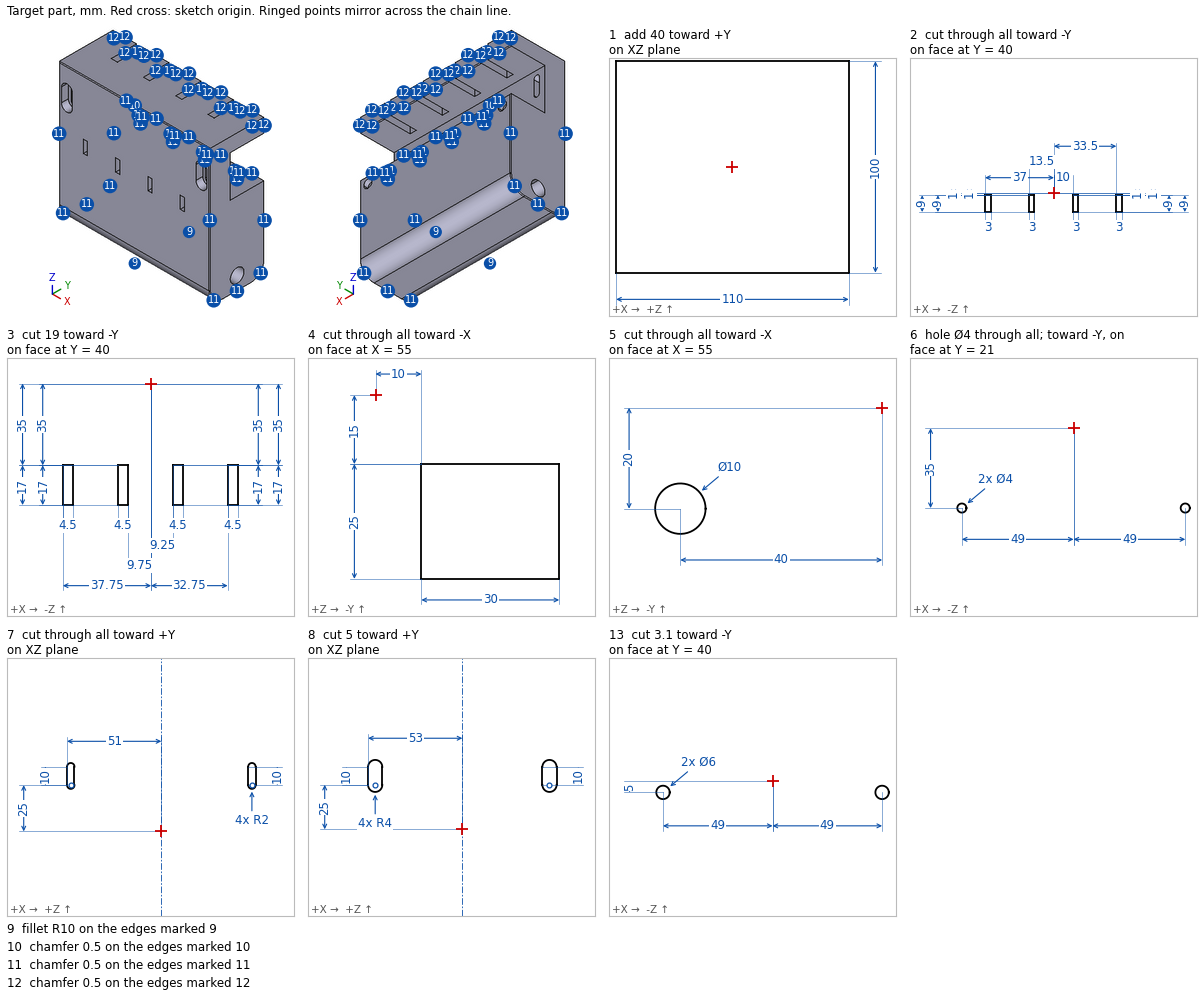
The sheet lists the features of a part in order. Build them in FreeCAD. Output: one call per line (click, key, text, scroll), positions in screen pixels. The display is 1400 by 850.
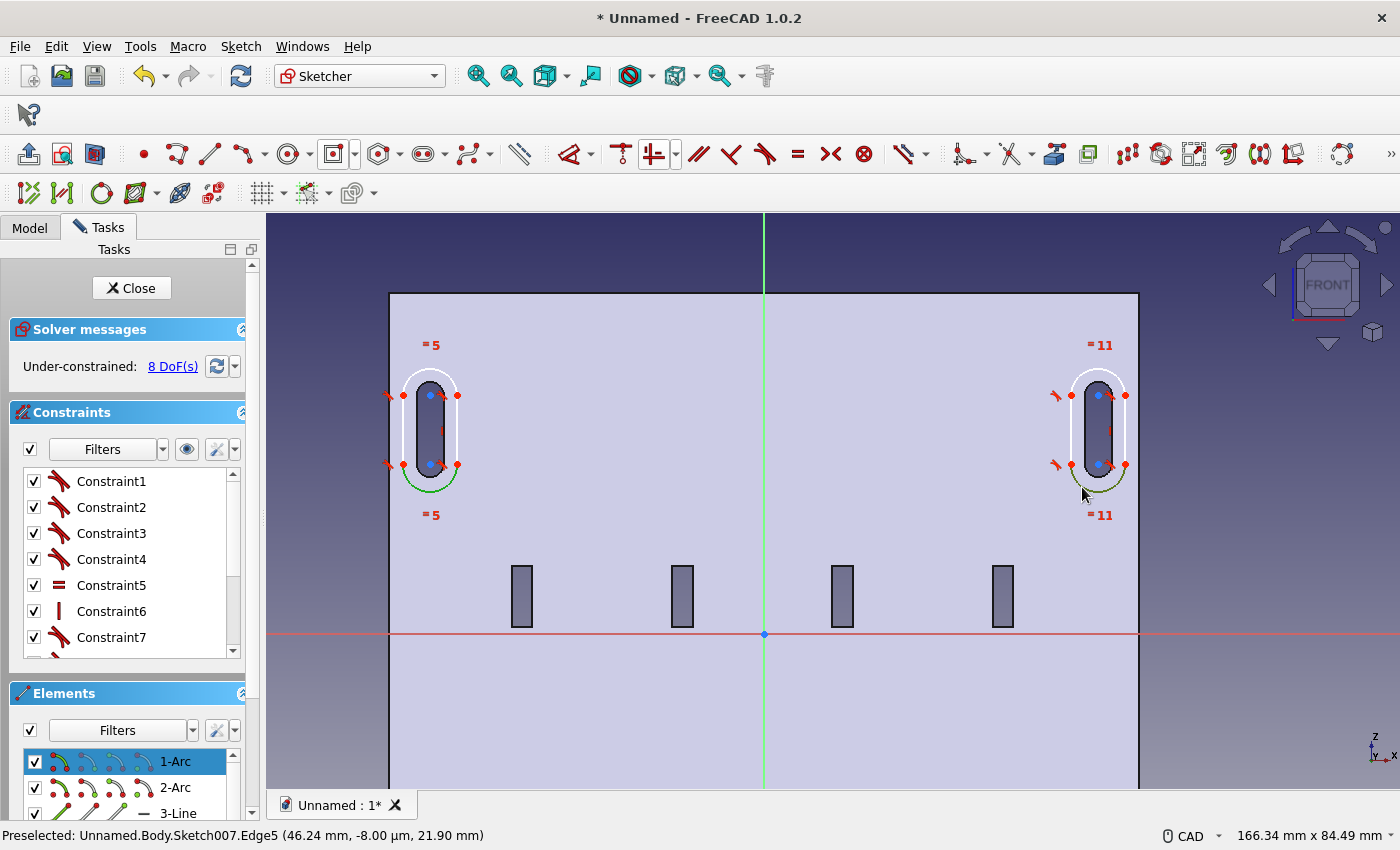
click(798, 154)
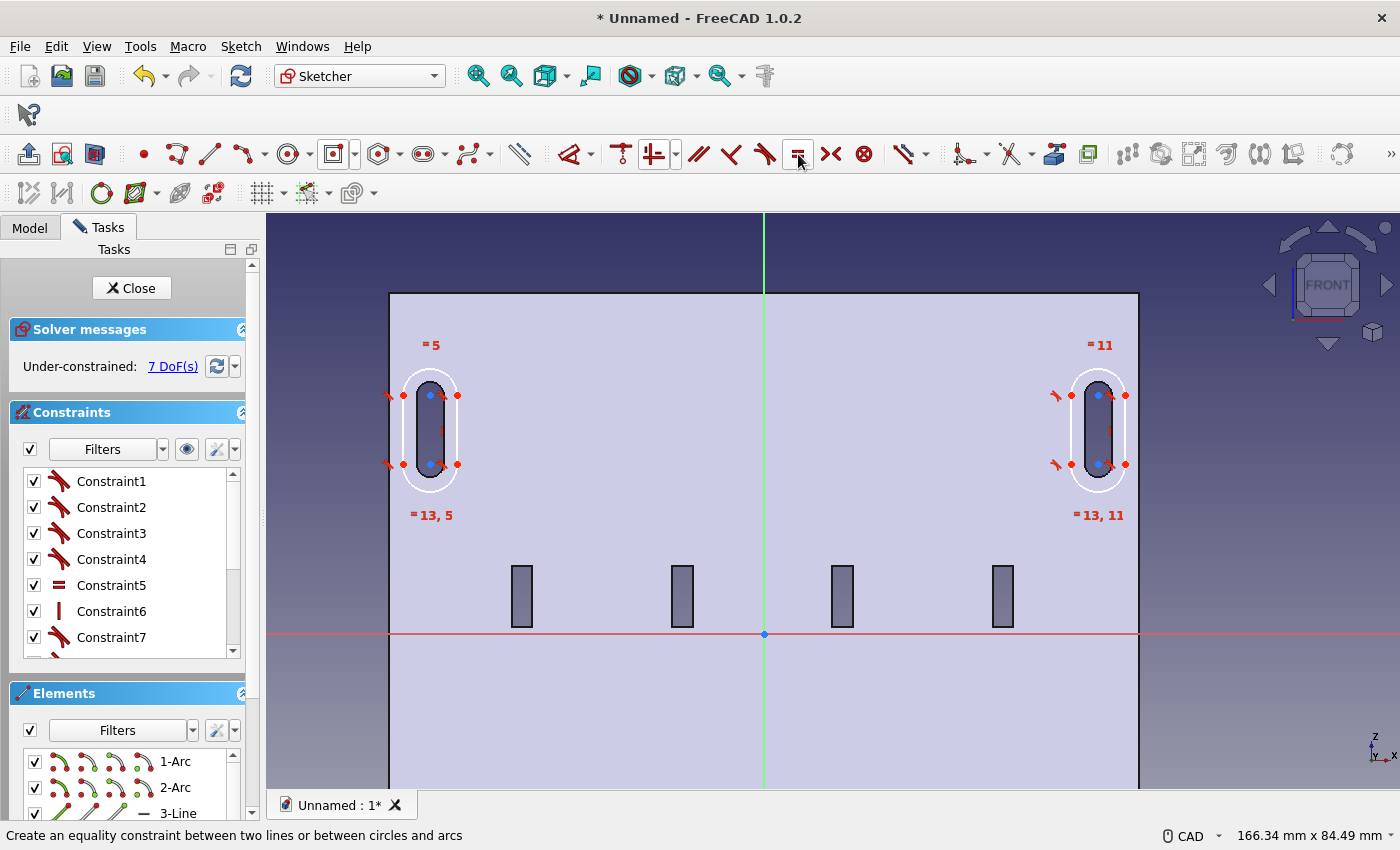
click(430, 465)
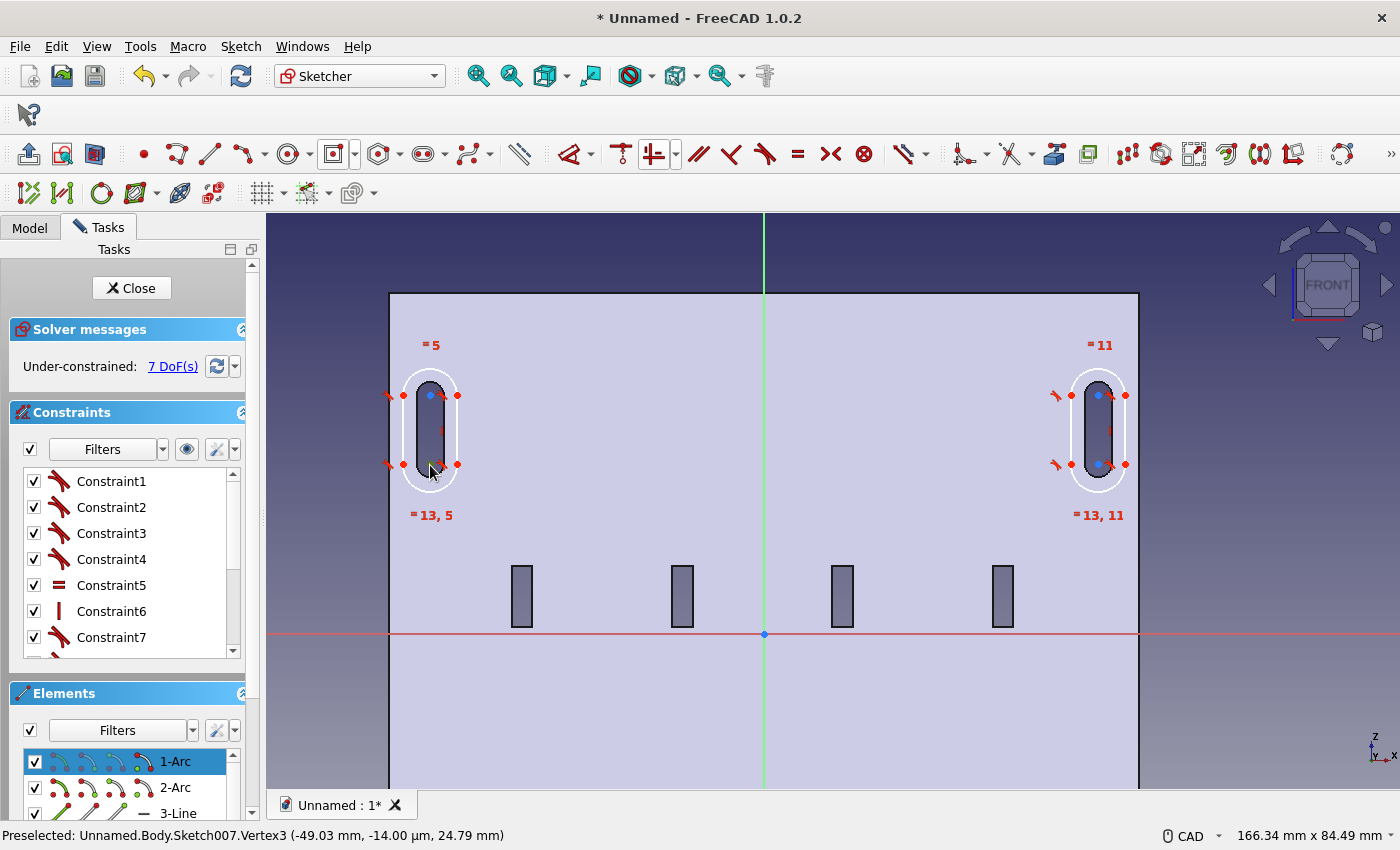
click(1098, 465)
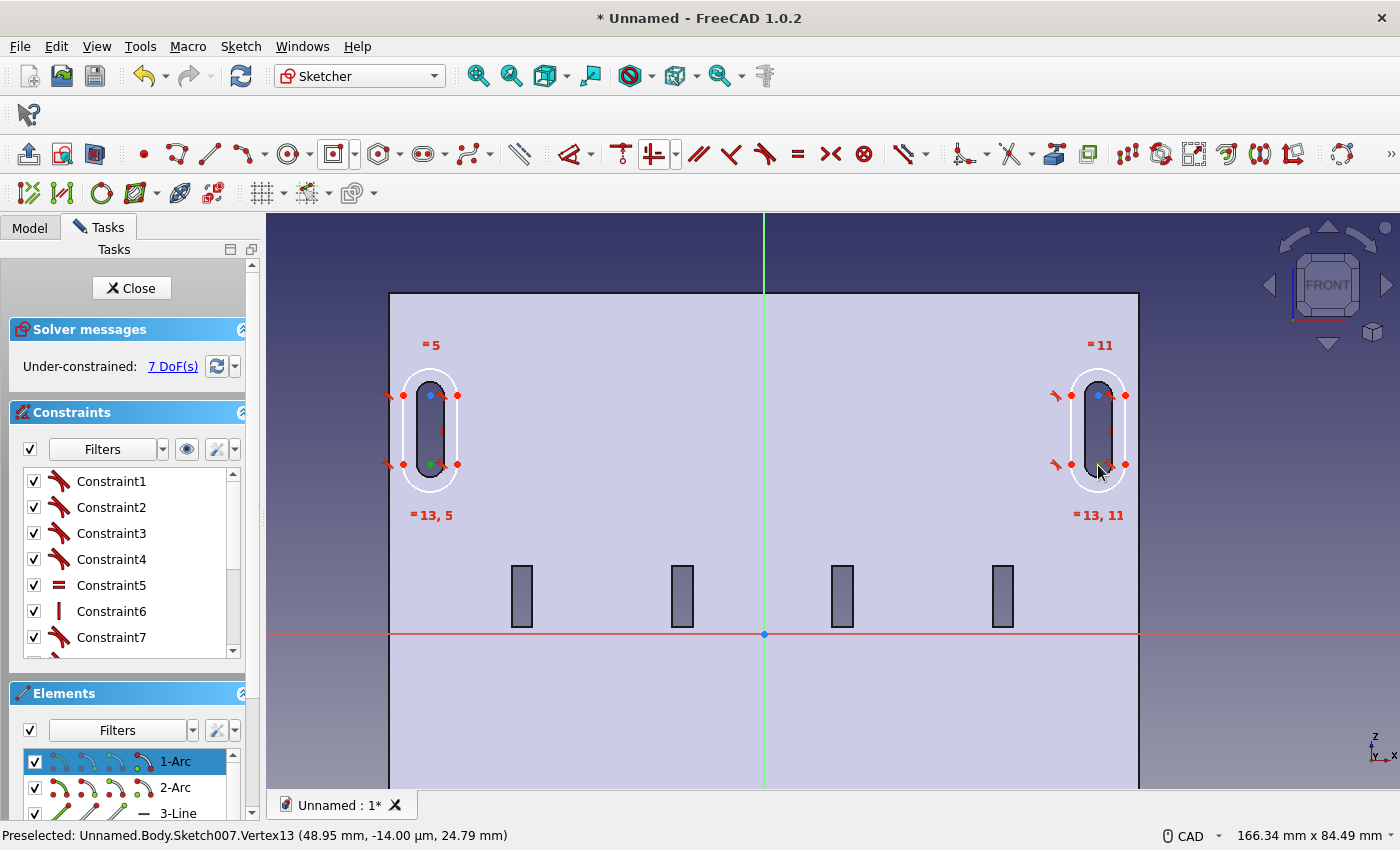
click(764, 724)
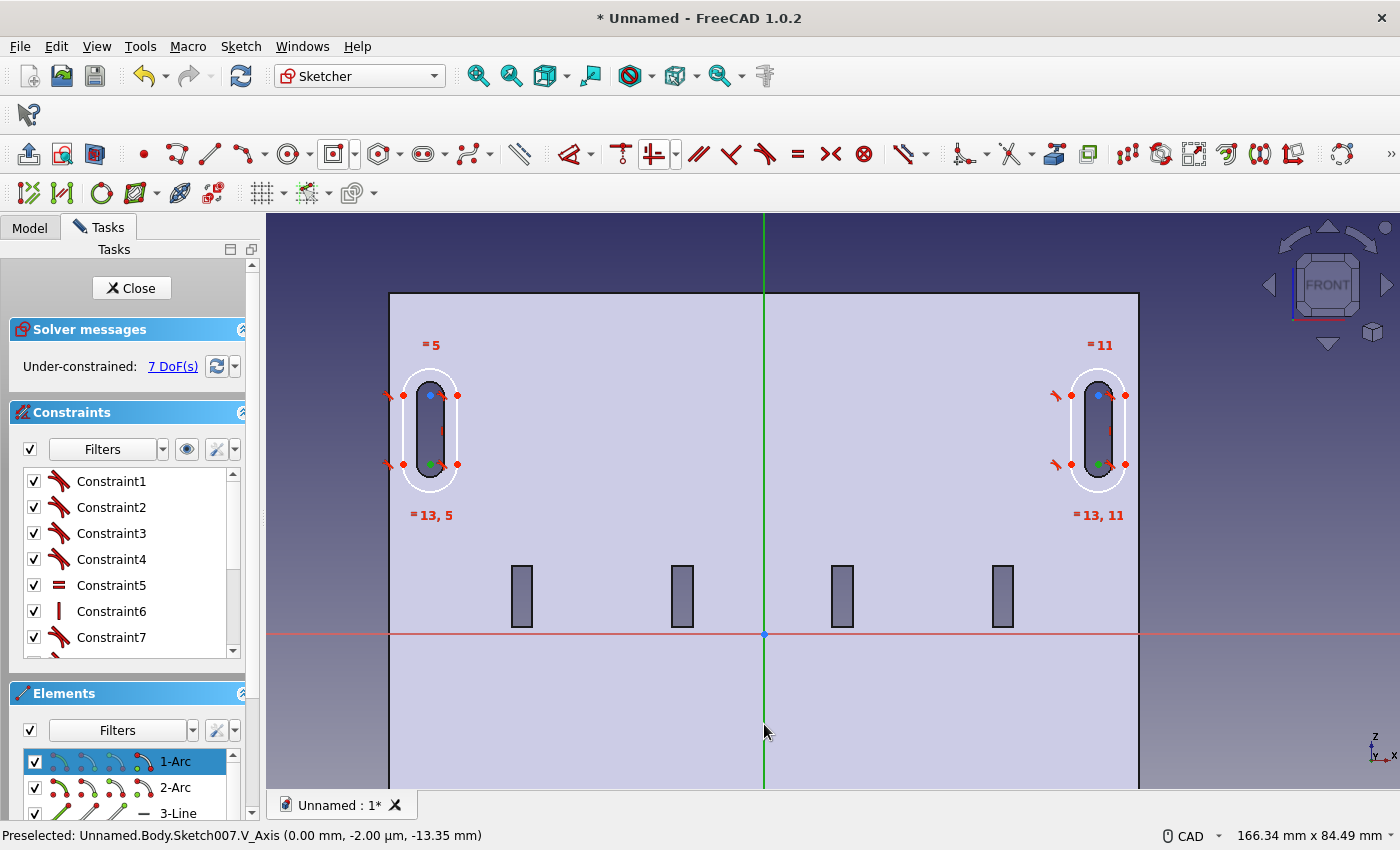
key(s)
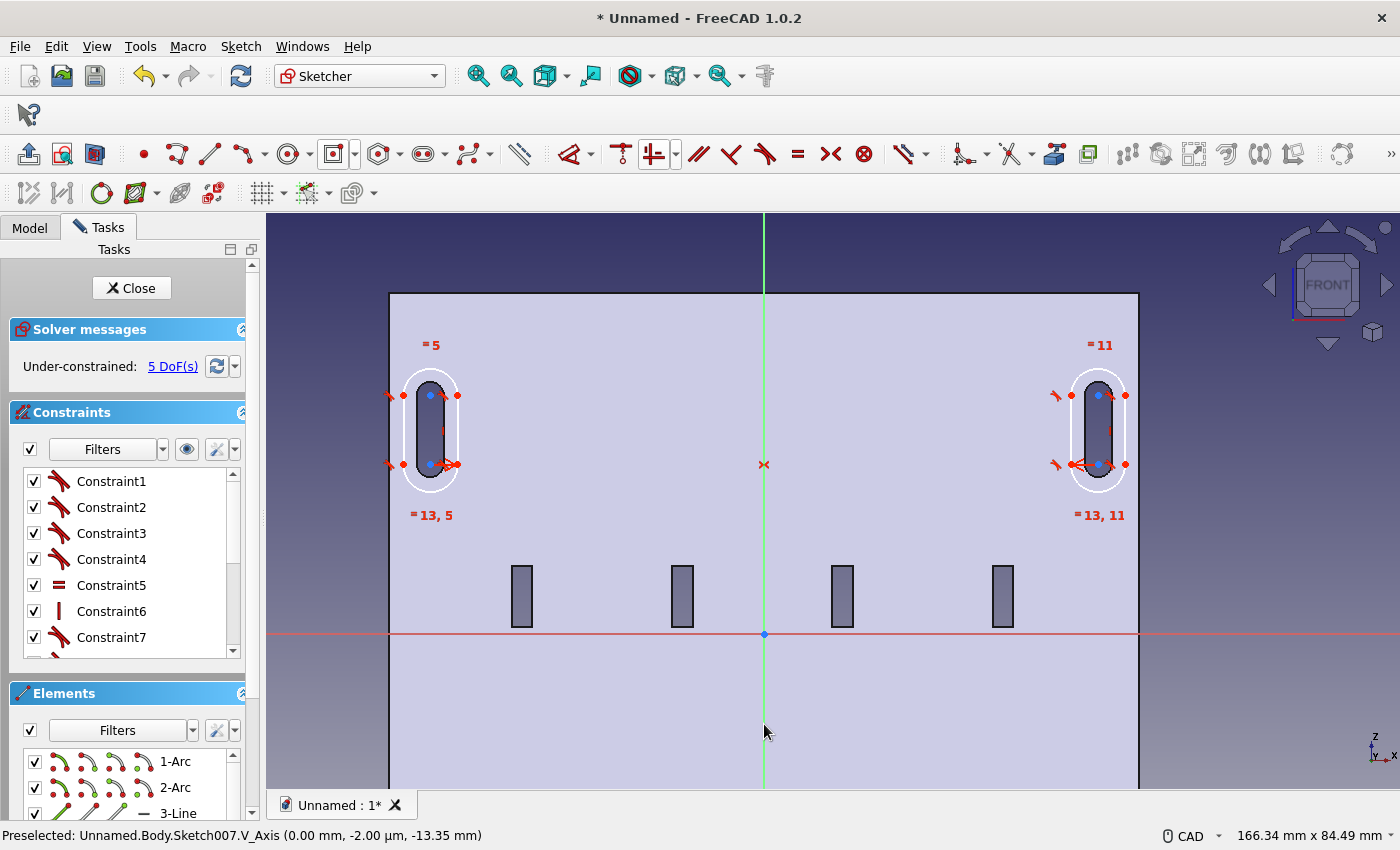
key(d)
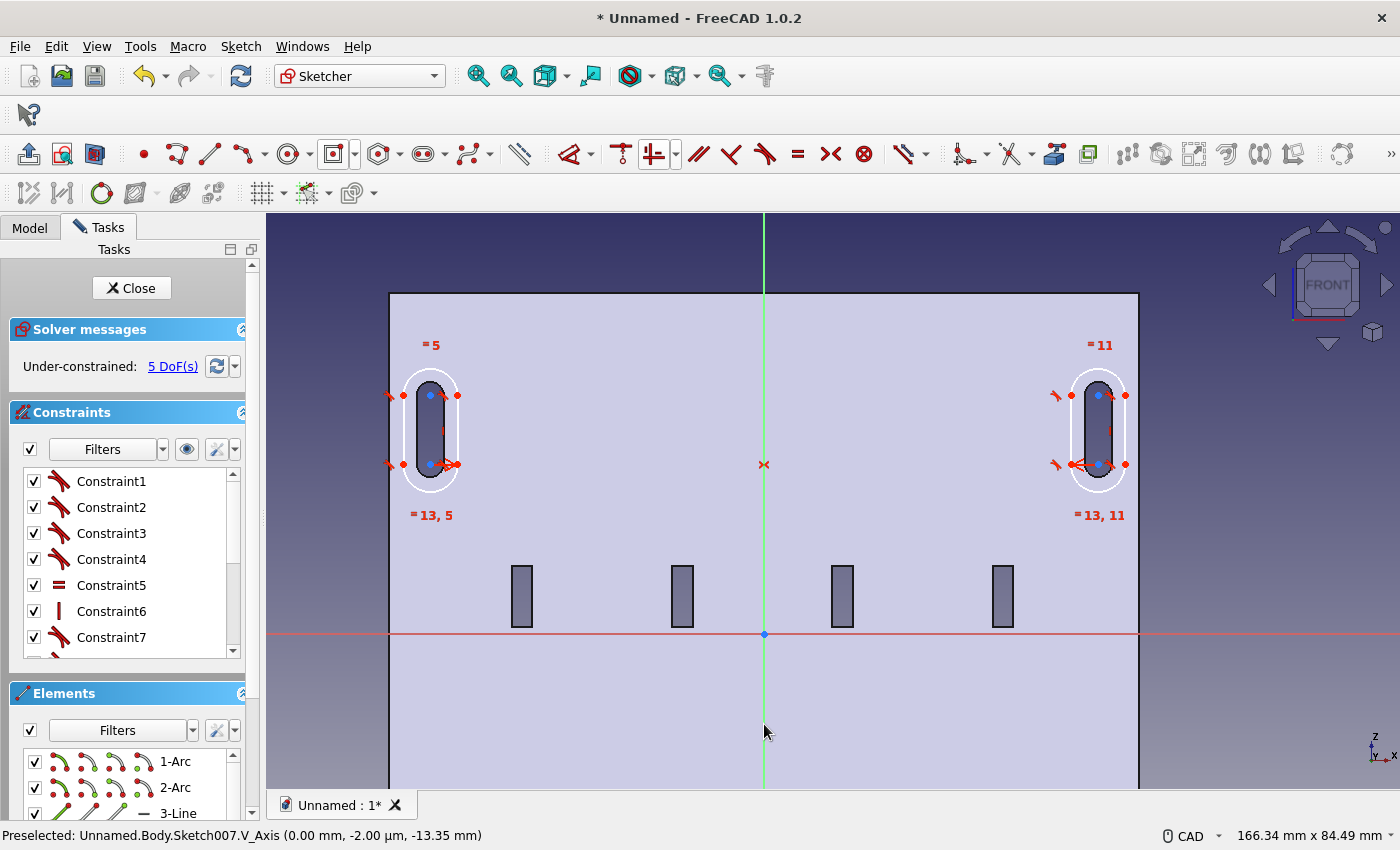
scroll(415, 487, up, 2)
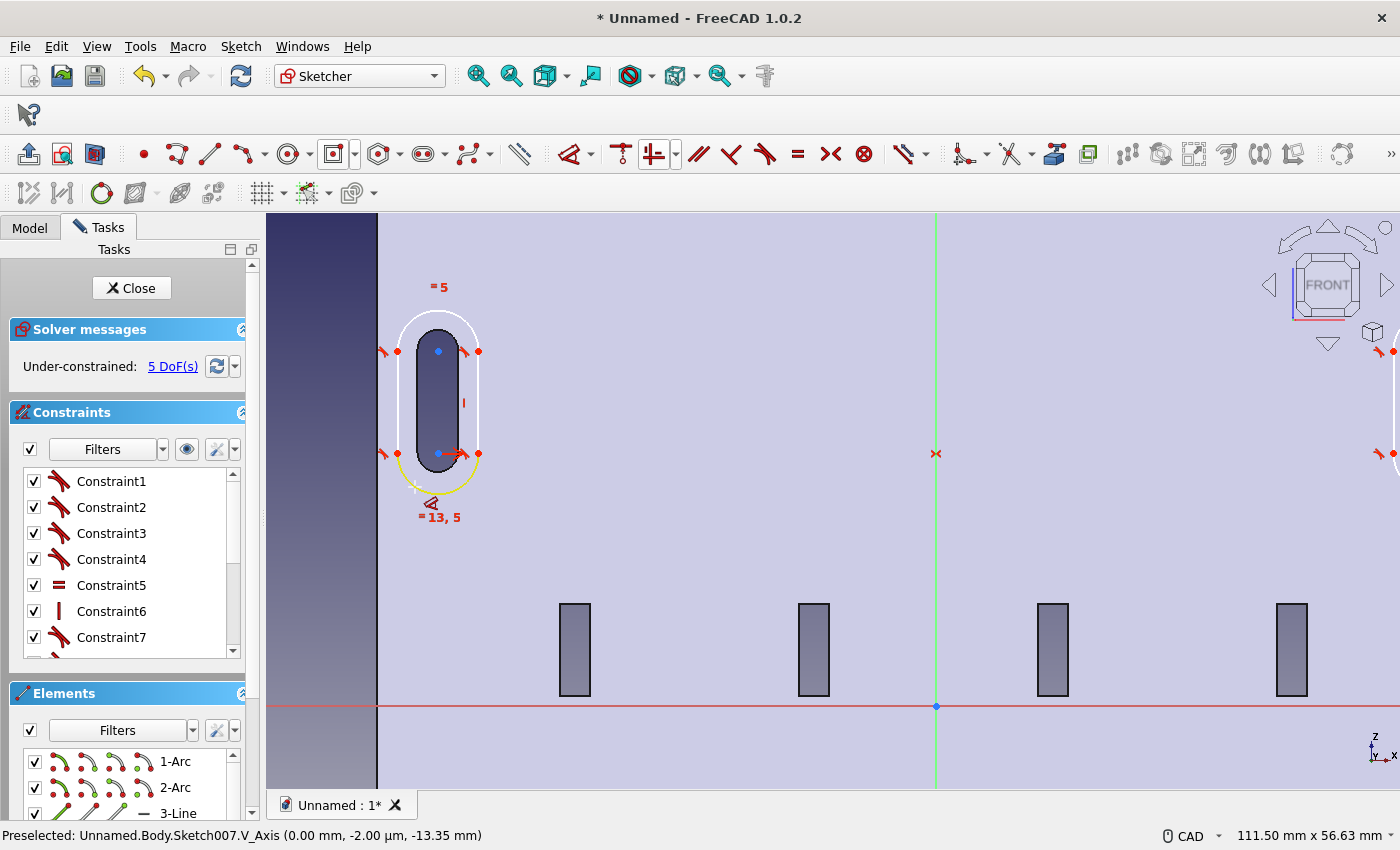
click(415, 487)
click(397, 513)